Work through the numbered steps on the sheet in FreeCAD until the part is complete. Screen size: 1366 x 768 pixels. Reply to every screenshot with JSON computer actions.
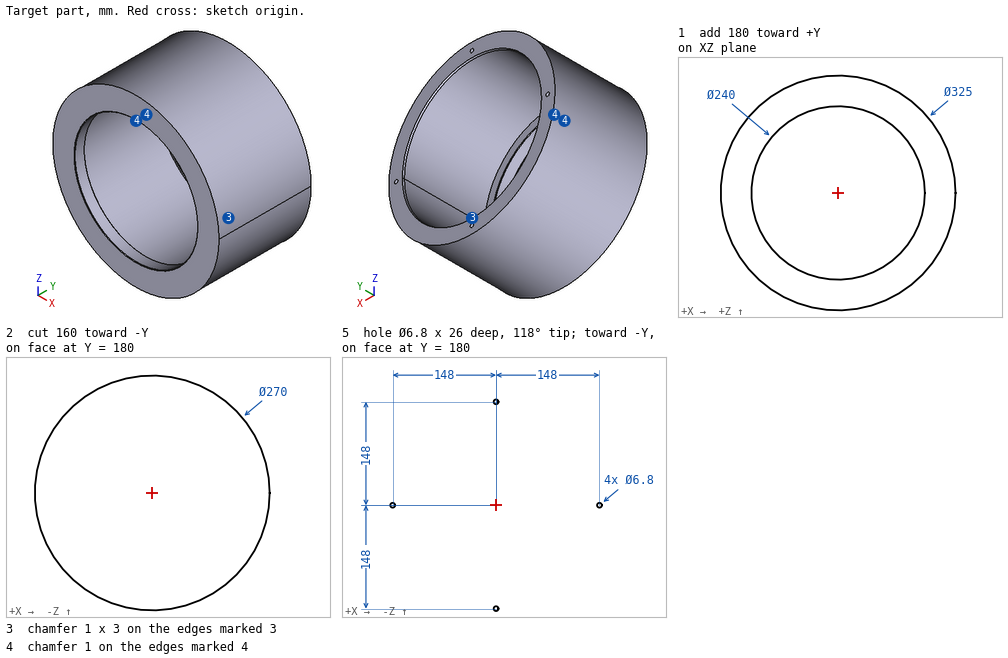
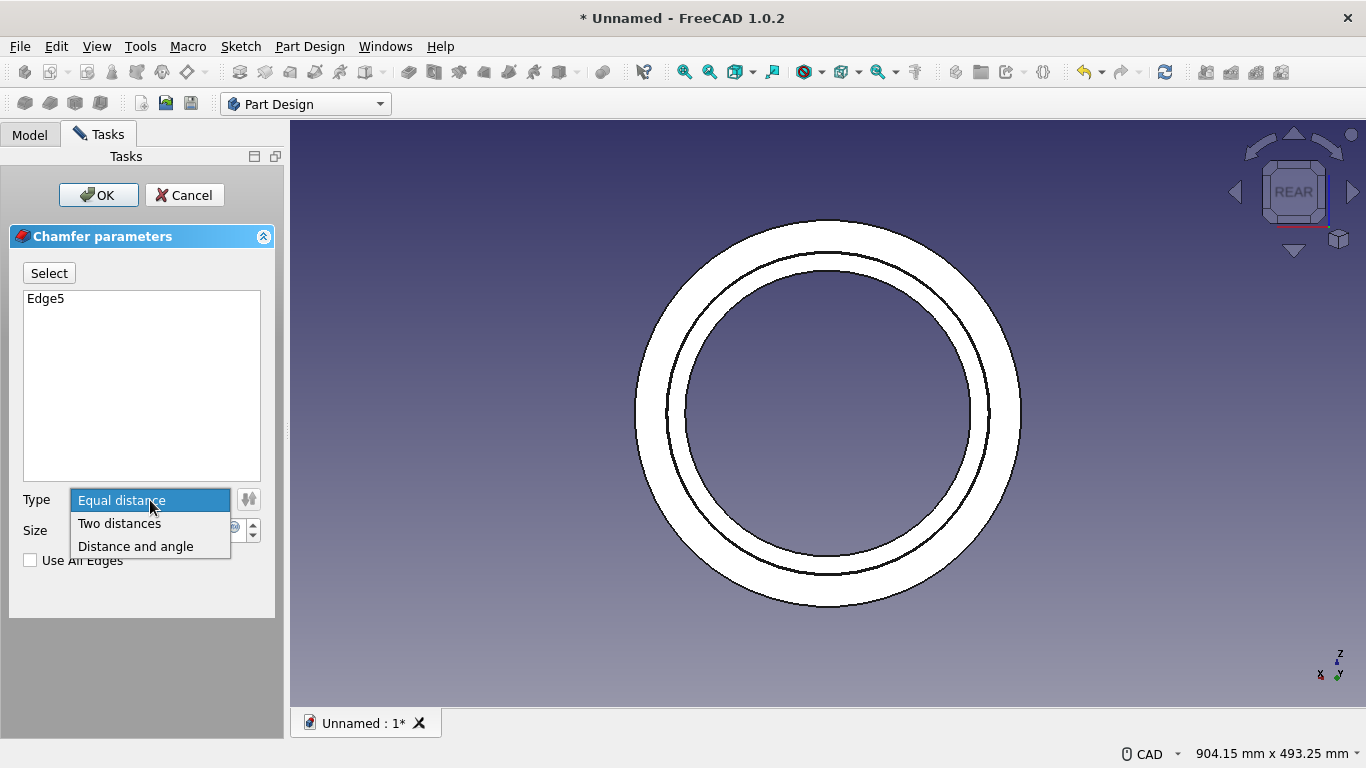
{"action": "left_click", "coordinate": [148, 524]}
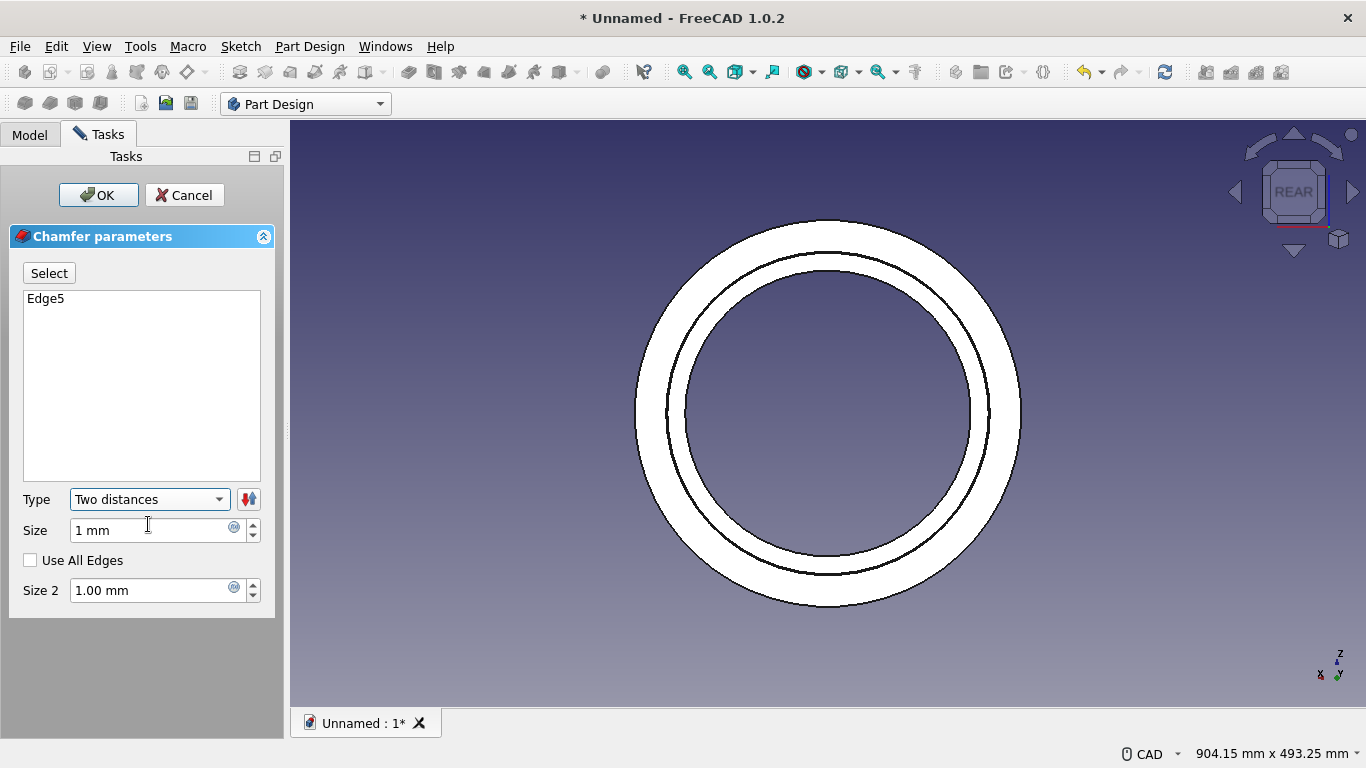
{"action": "triple_click", "coordinate": [158, 590]}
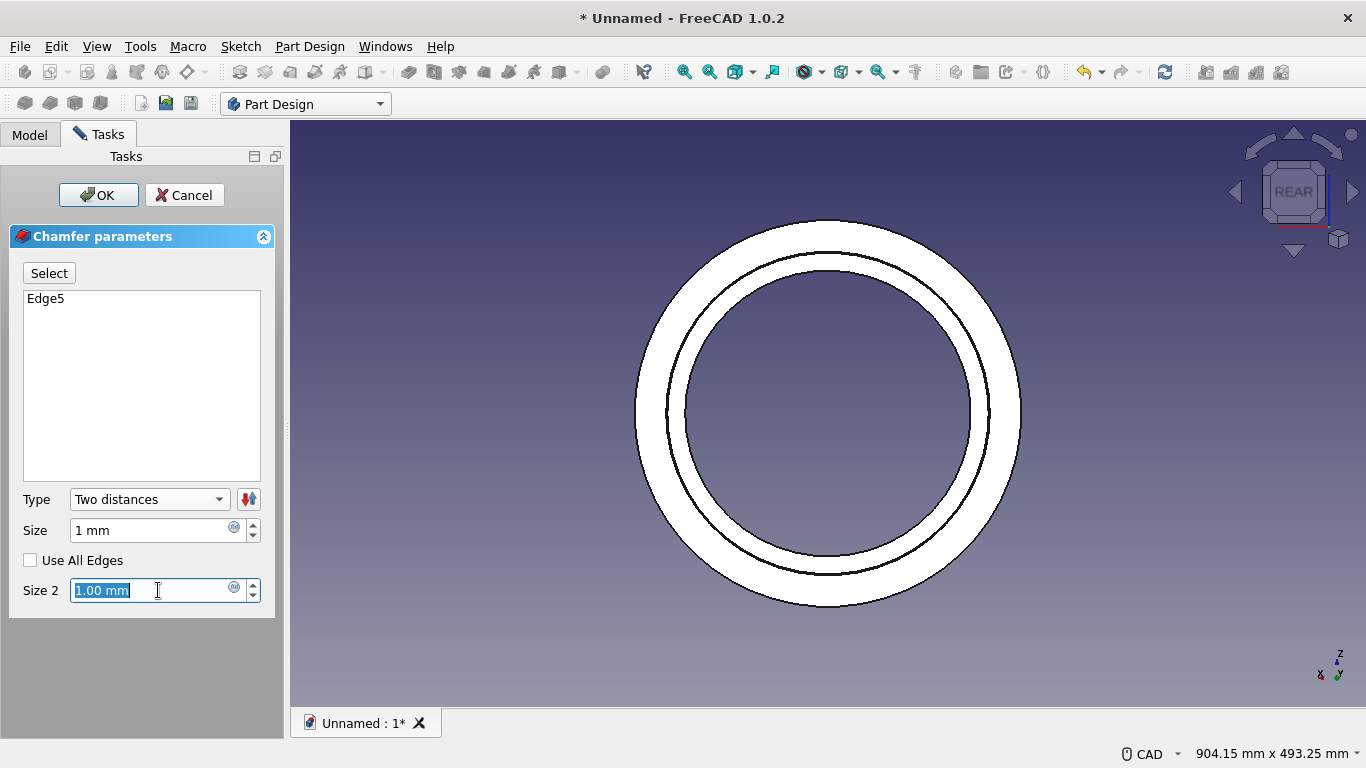
{"action": "type", "text": "3"}
{"action": "key", "text": "Tab"}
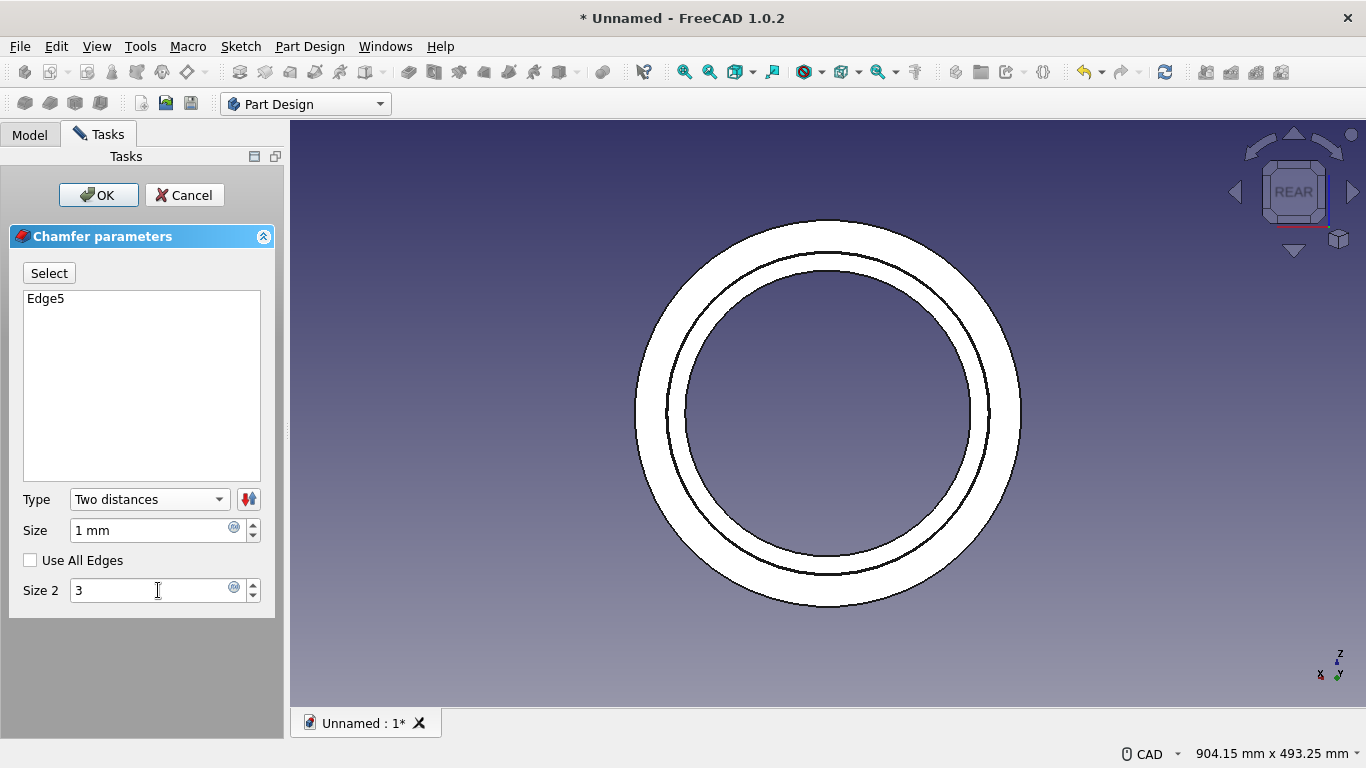
{"action": "left_click", "coordinate": [99, 195]}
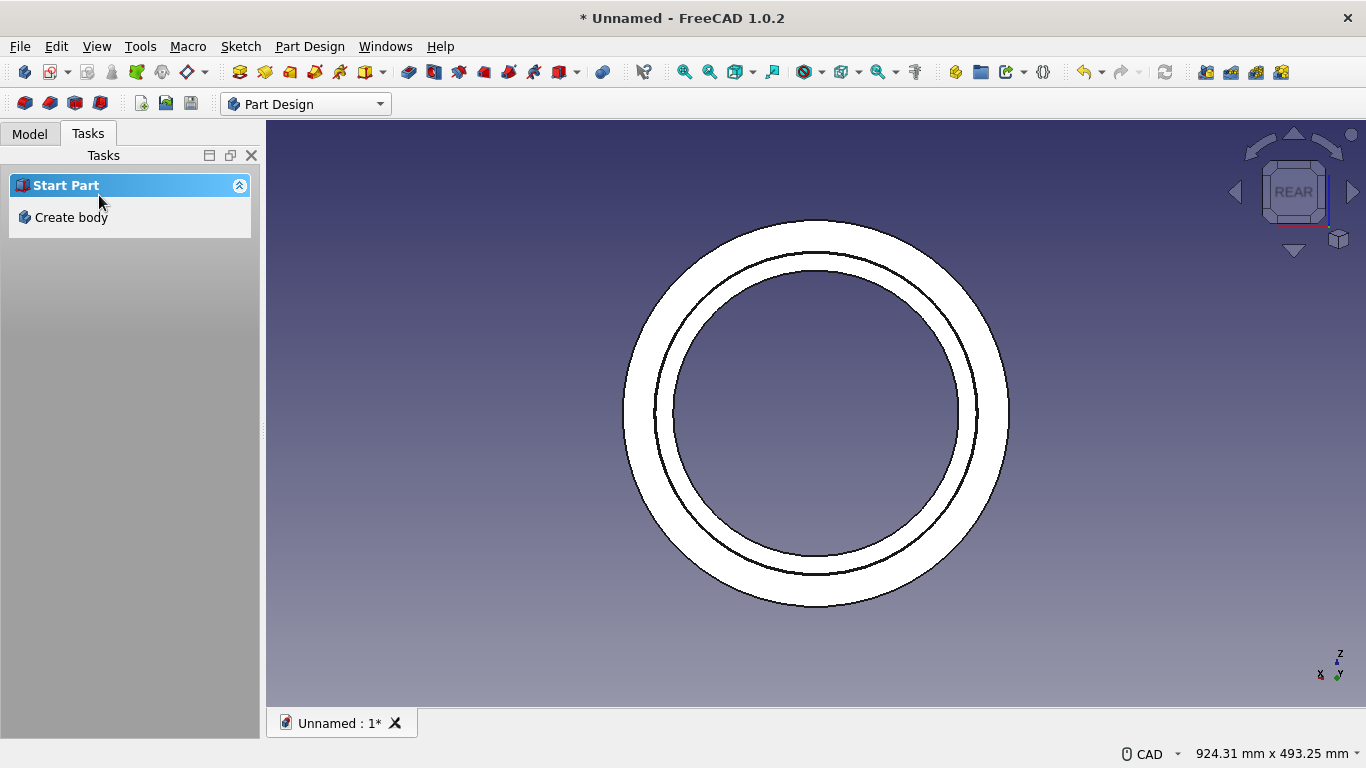
{"action": "left_click", "coordinate": [932, 329]}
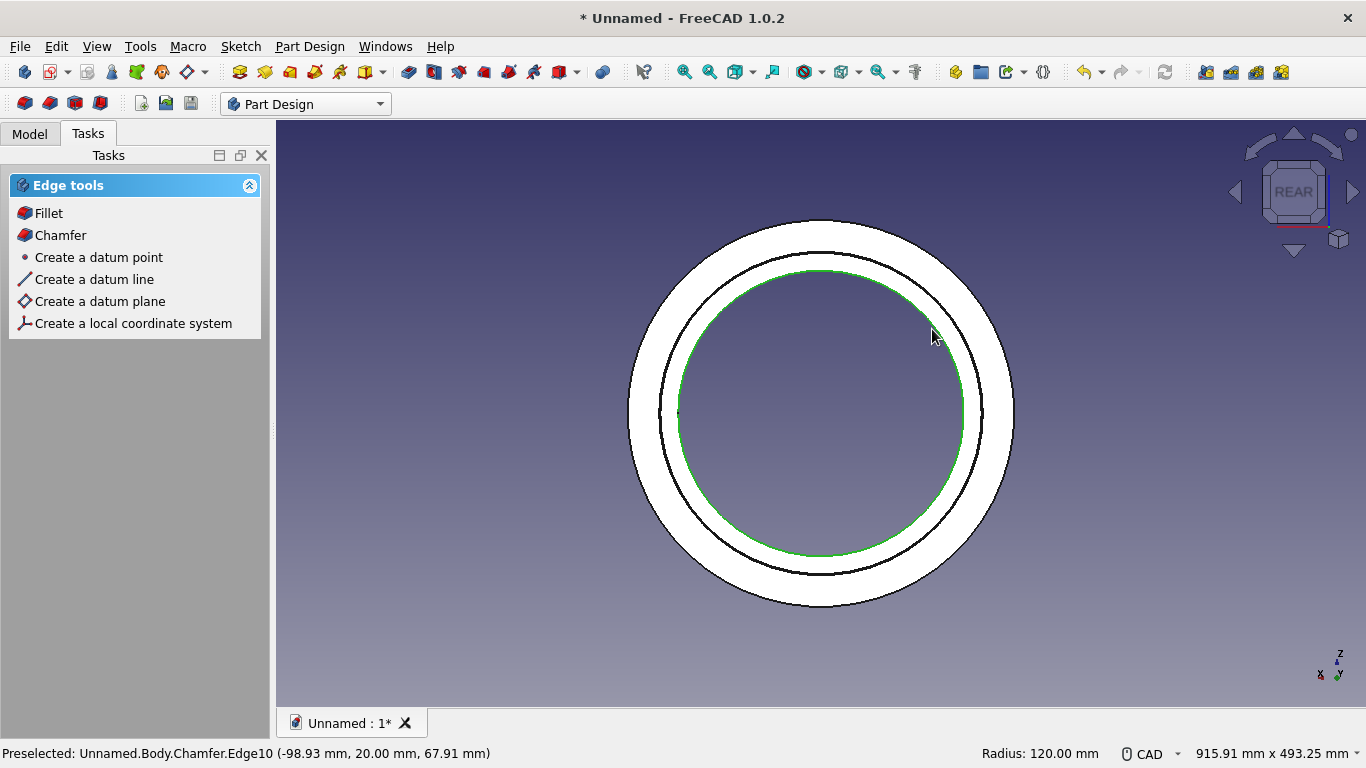
{"action": "key", "text": "0"}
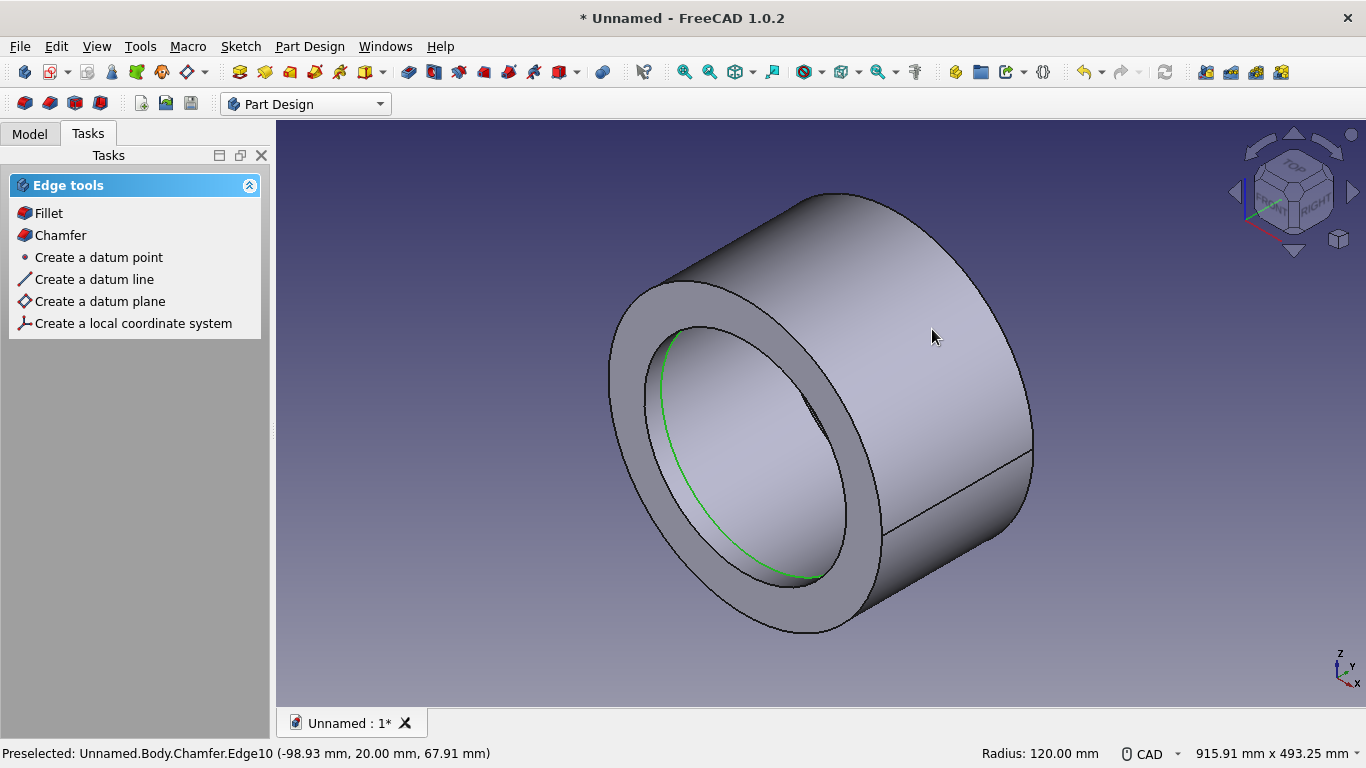
{"action": "left_click", "coordinate": [644, 398], "text": "ctrl"}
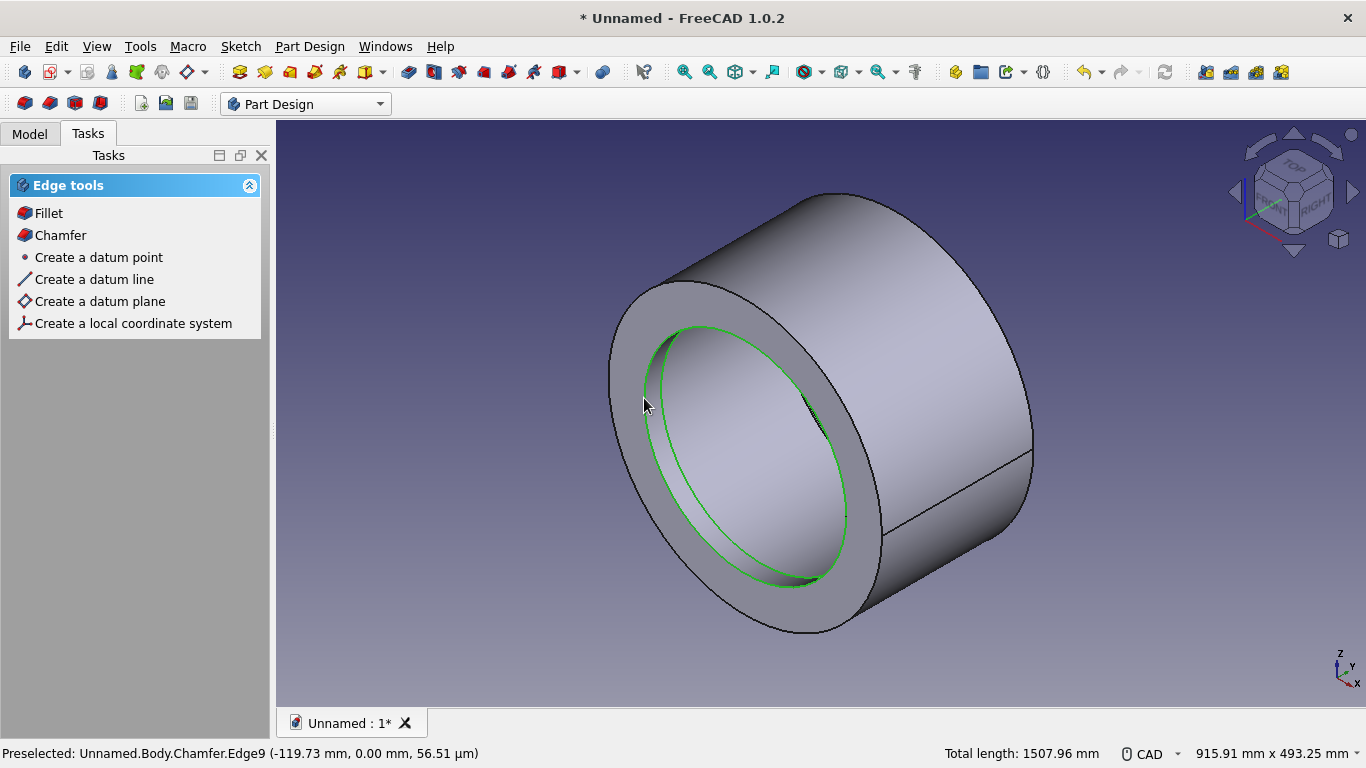
{"action": "left_click", "coordinate": [50, 104]}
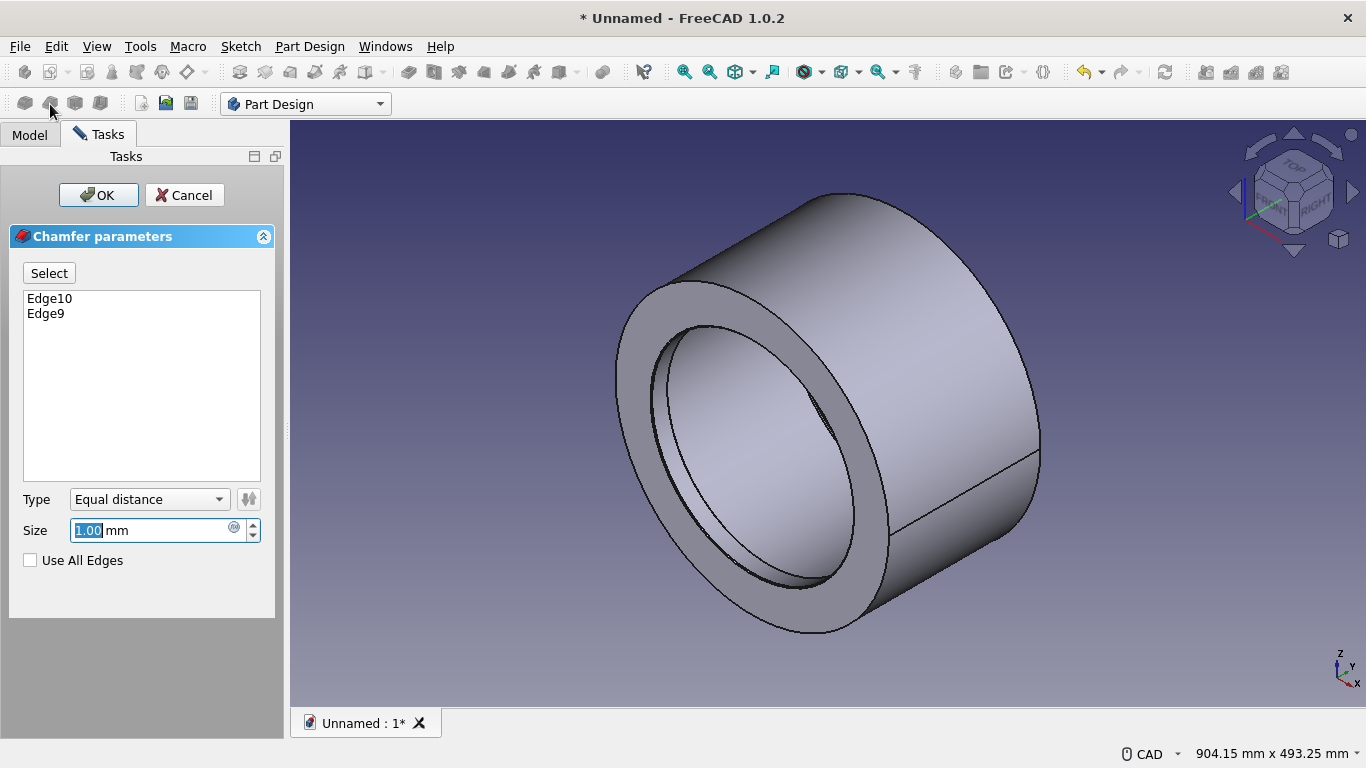
{"action": "type", "text": "1"}
{"action": "key", "text": "Tab"}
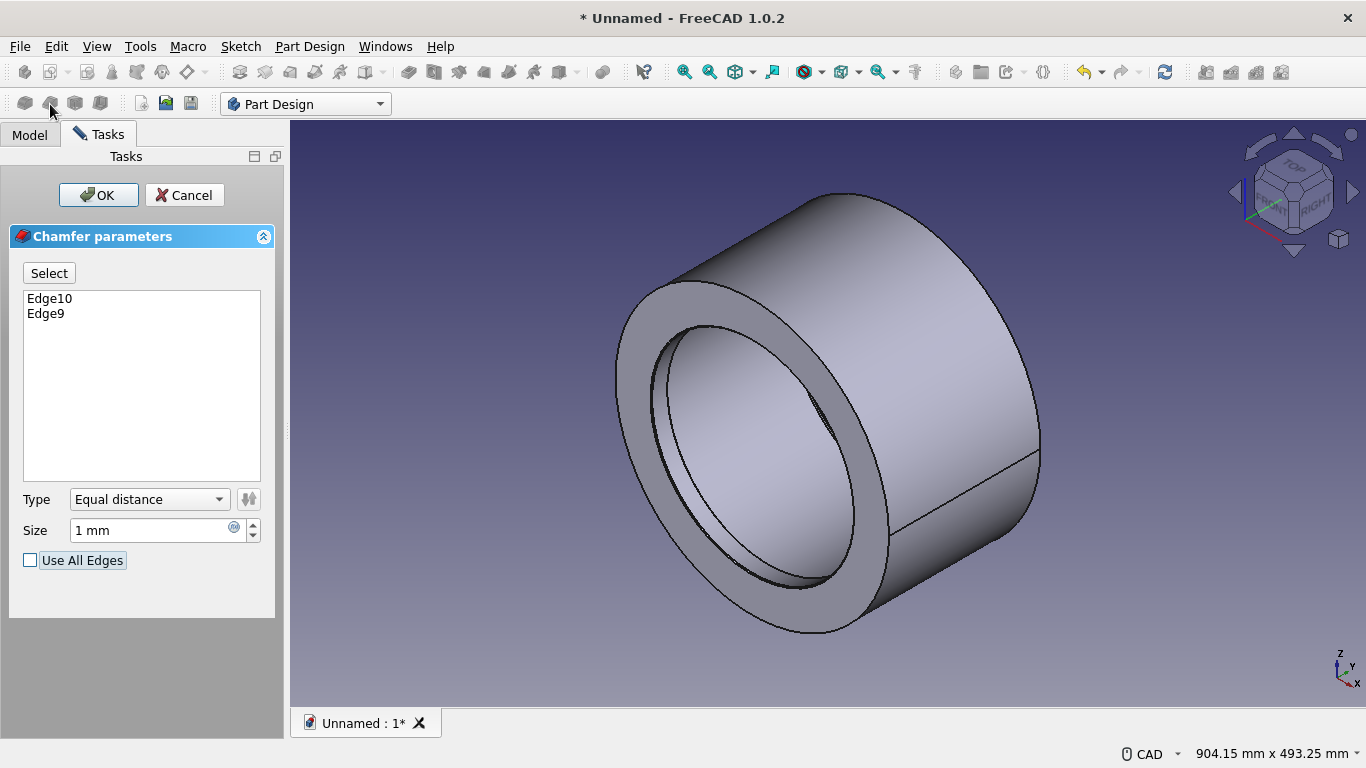
{"action": "left_click", "coordinate": [99, 195]}